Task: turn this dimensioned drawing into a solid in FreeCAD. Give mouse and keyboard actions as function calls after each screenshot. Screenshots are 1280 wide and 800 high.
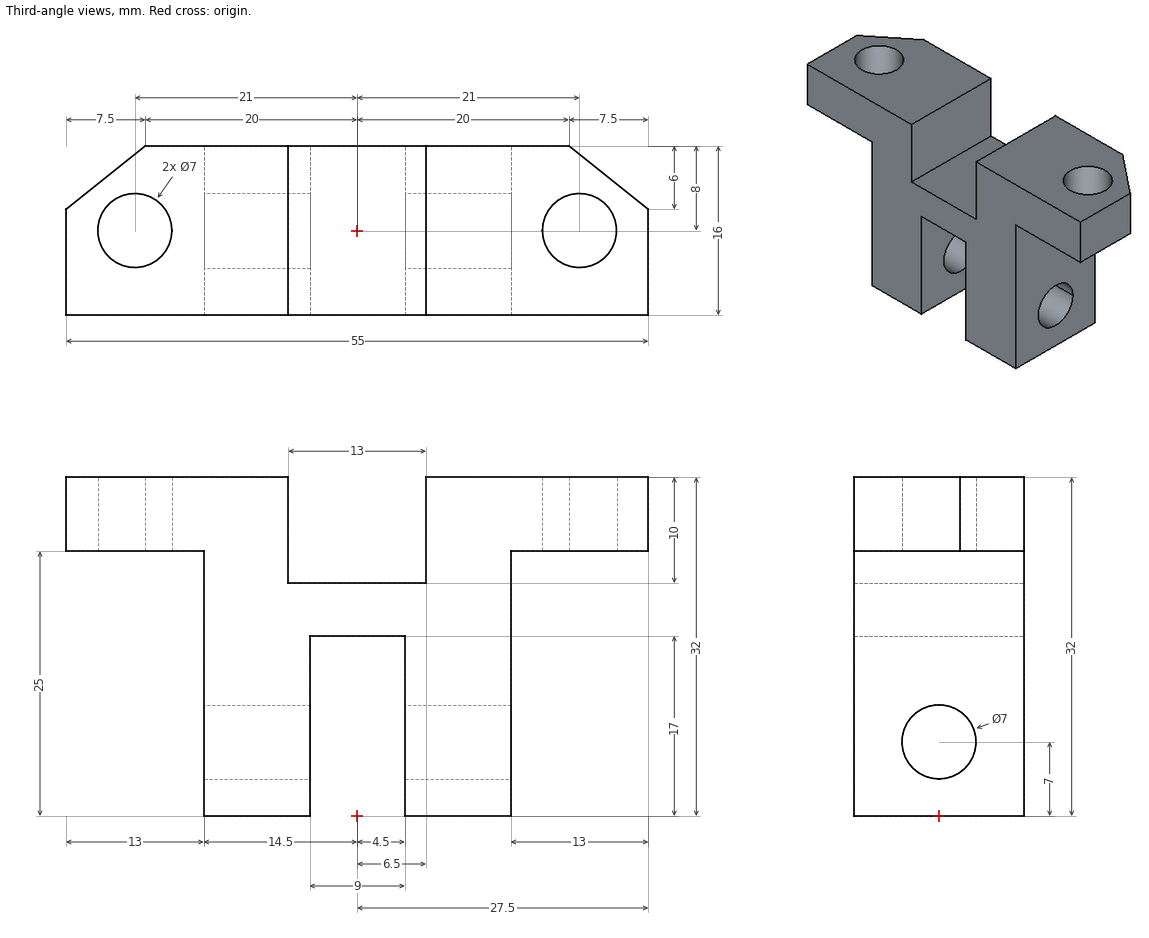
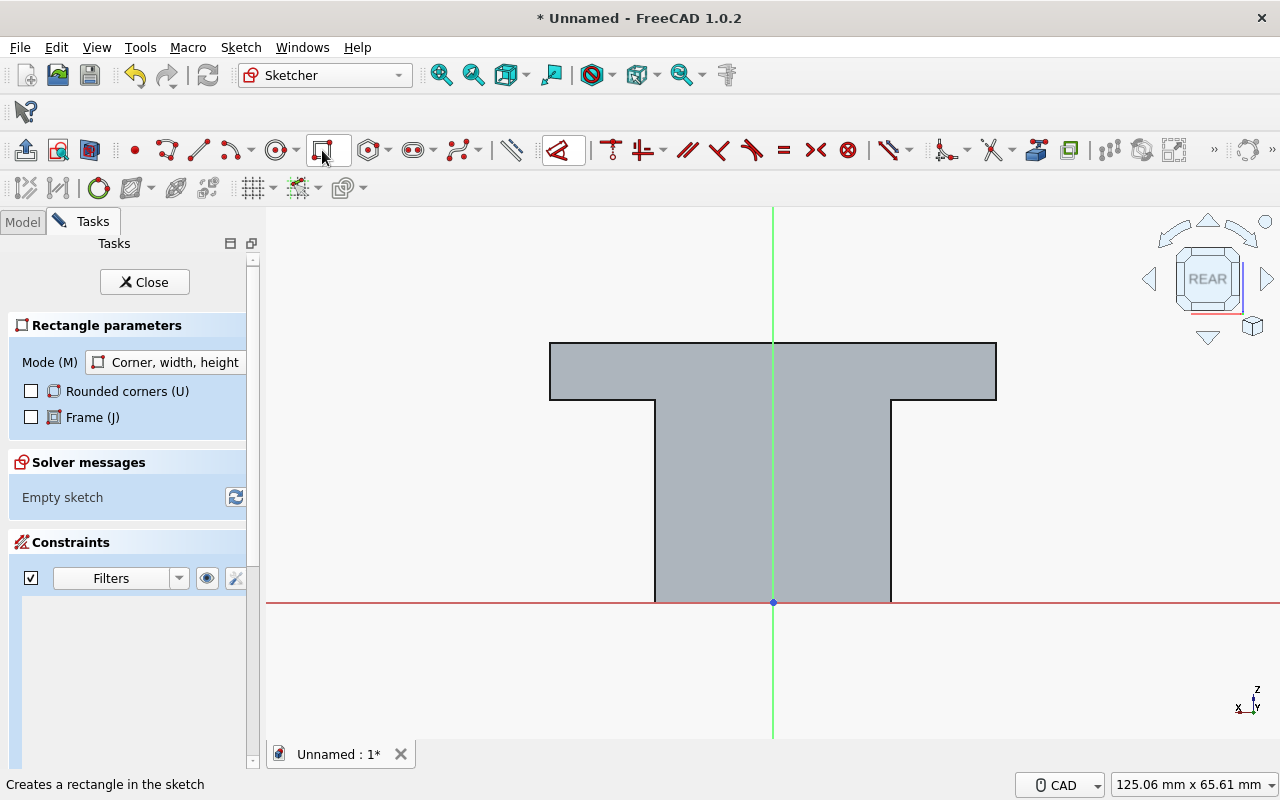
click(720, 343)
click(826, 424)
key(Escape)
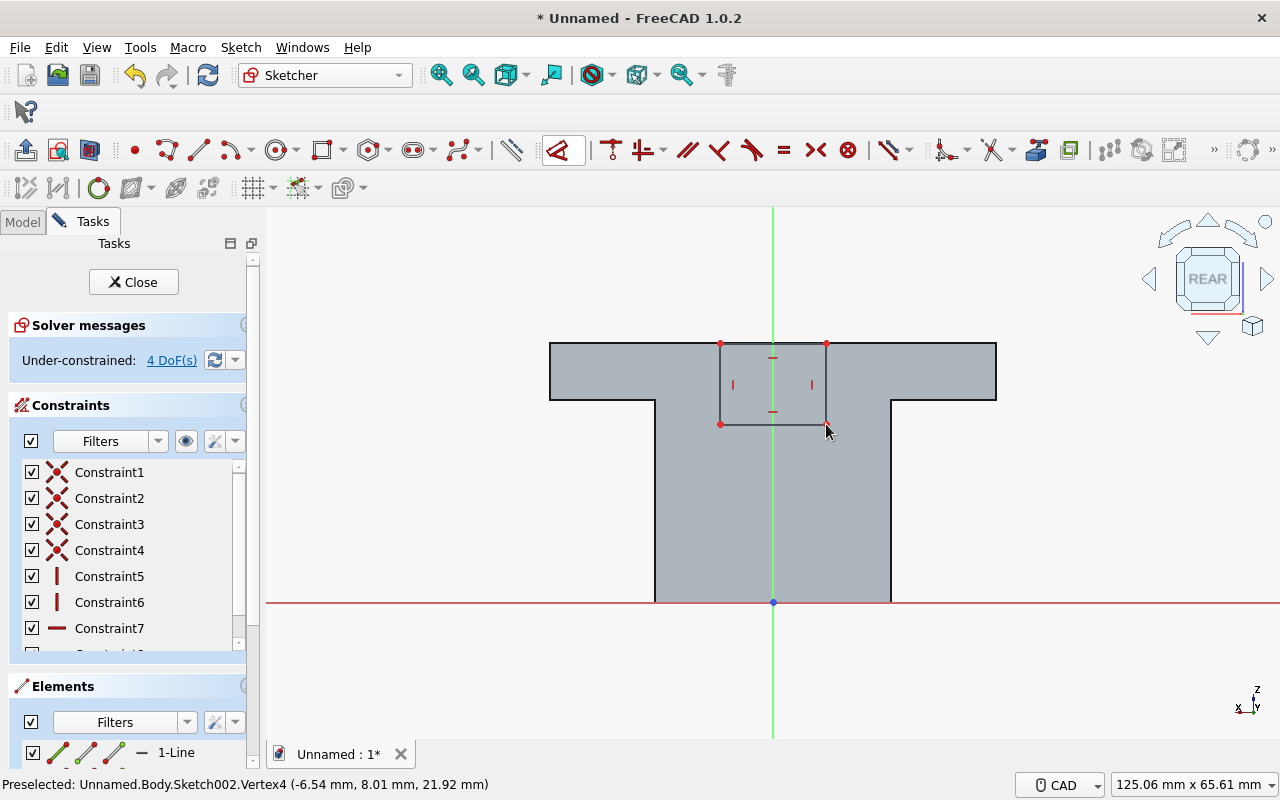
click(720, 368)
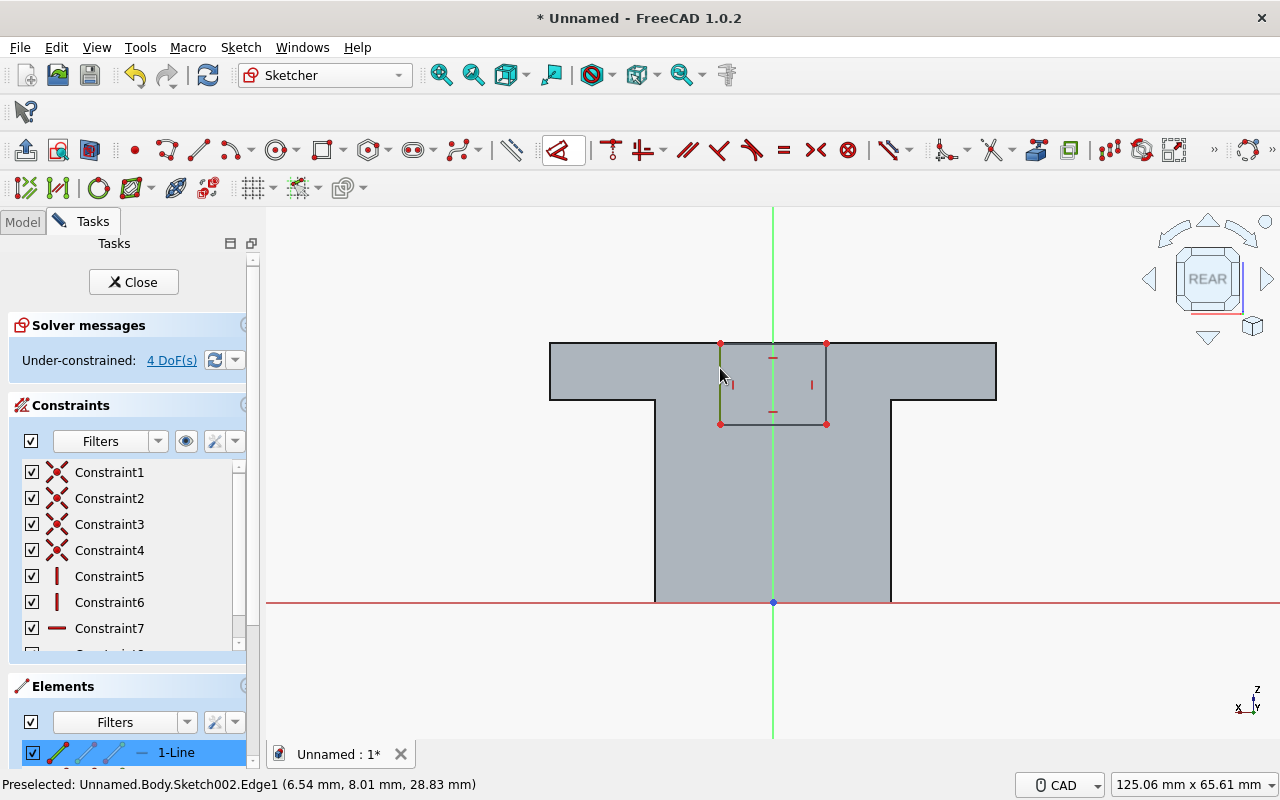
key(i)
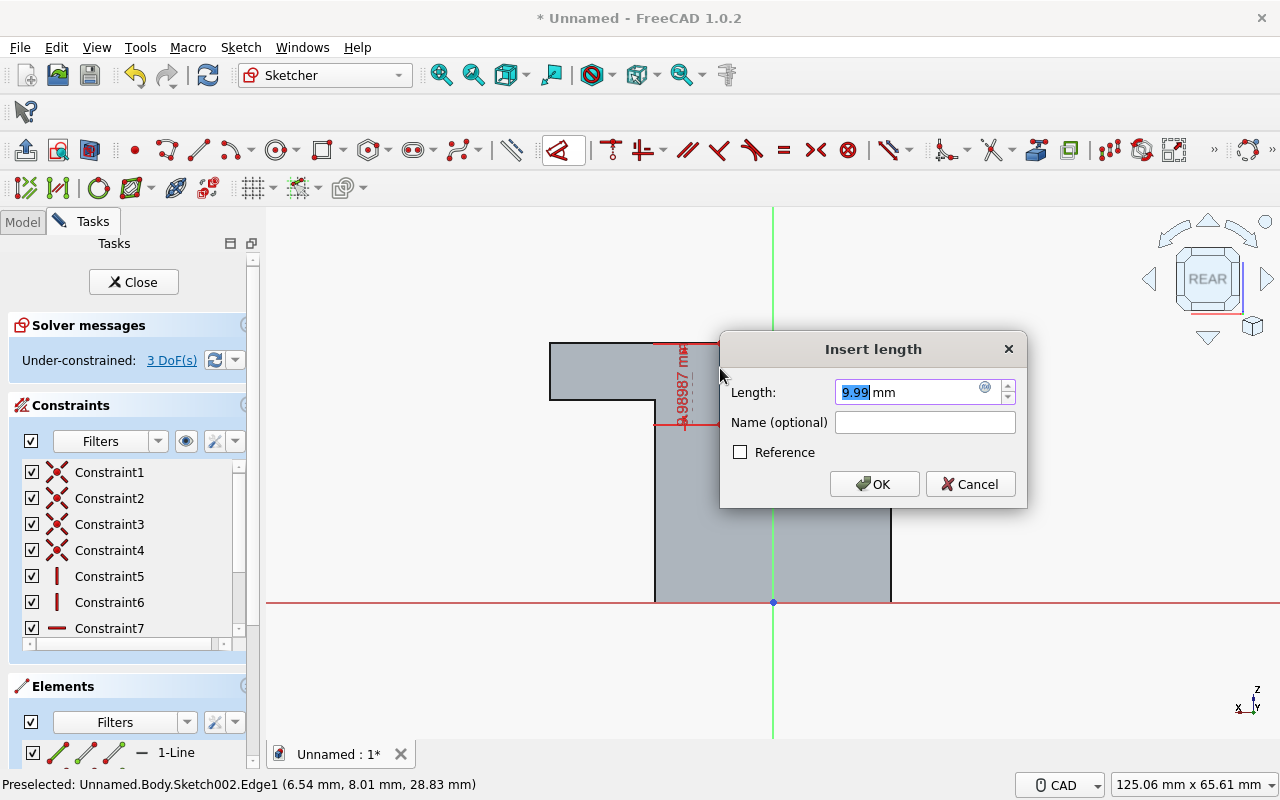
text(10)
key(Return)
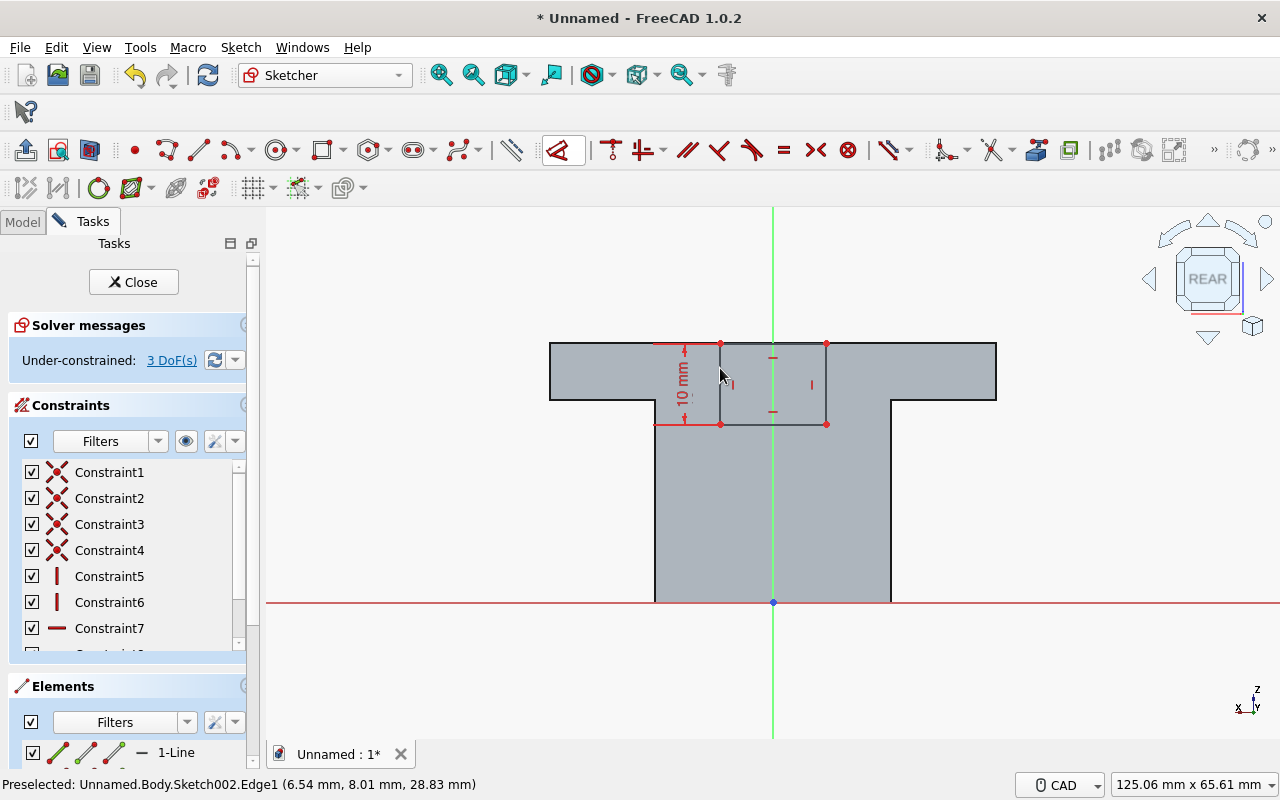
click(752, 425)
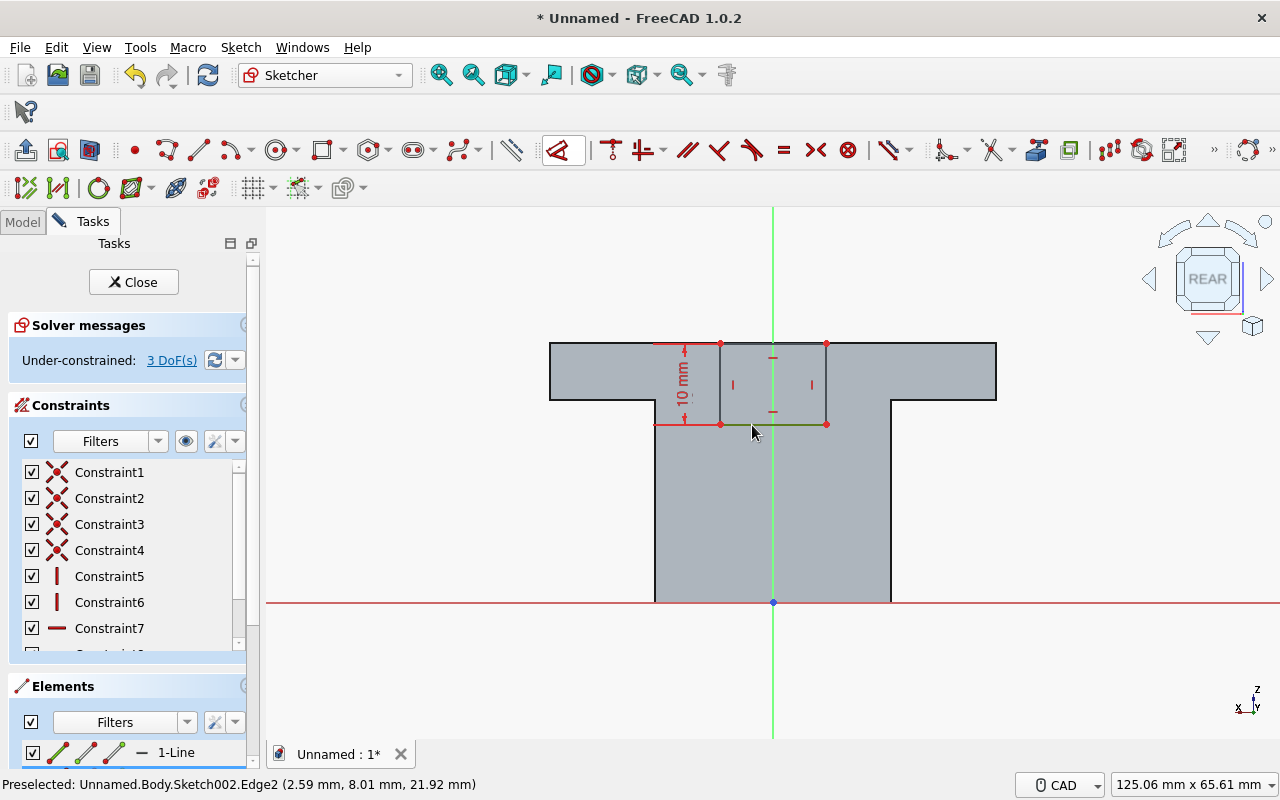
click(580, 150)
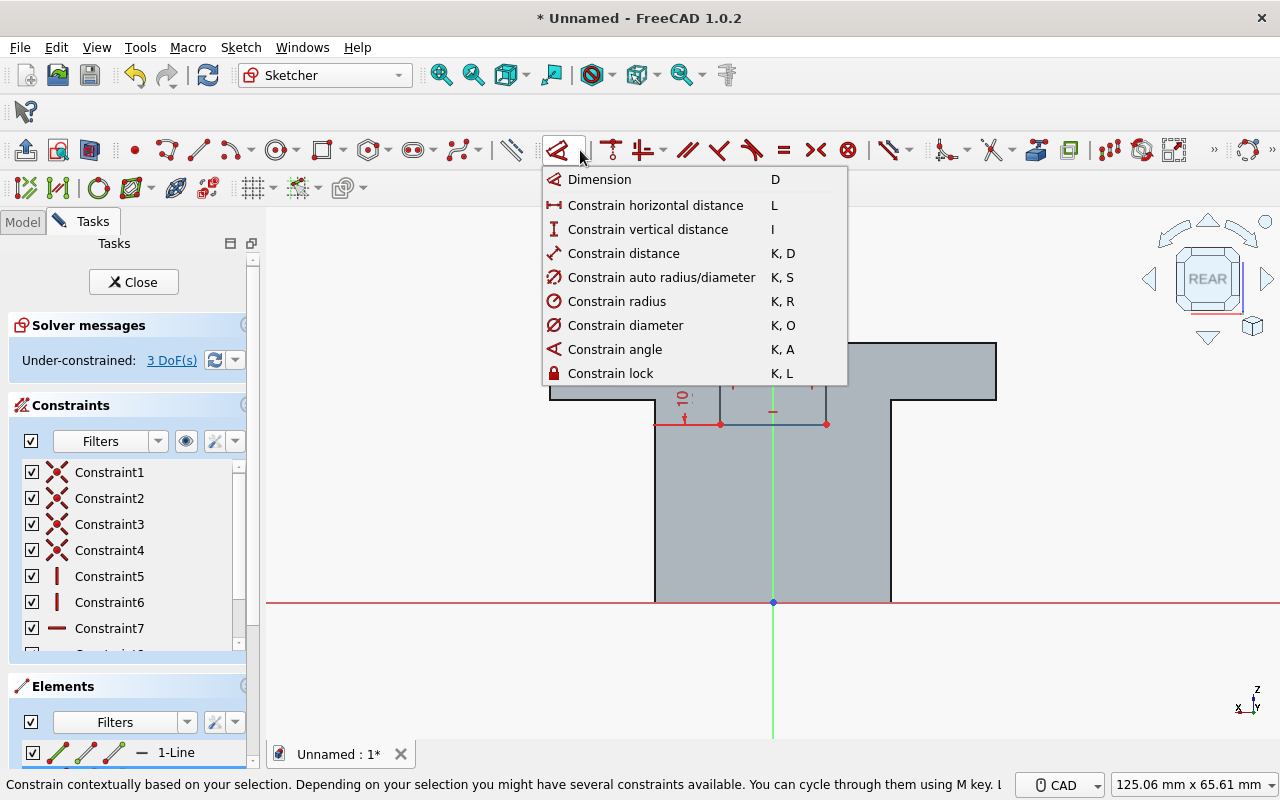
click(695, 205)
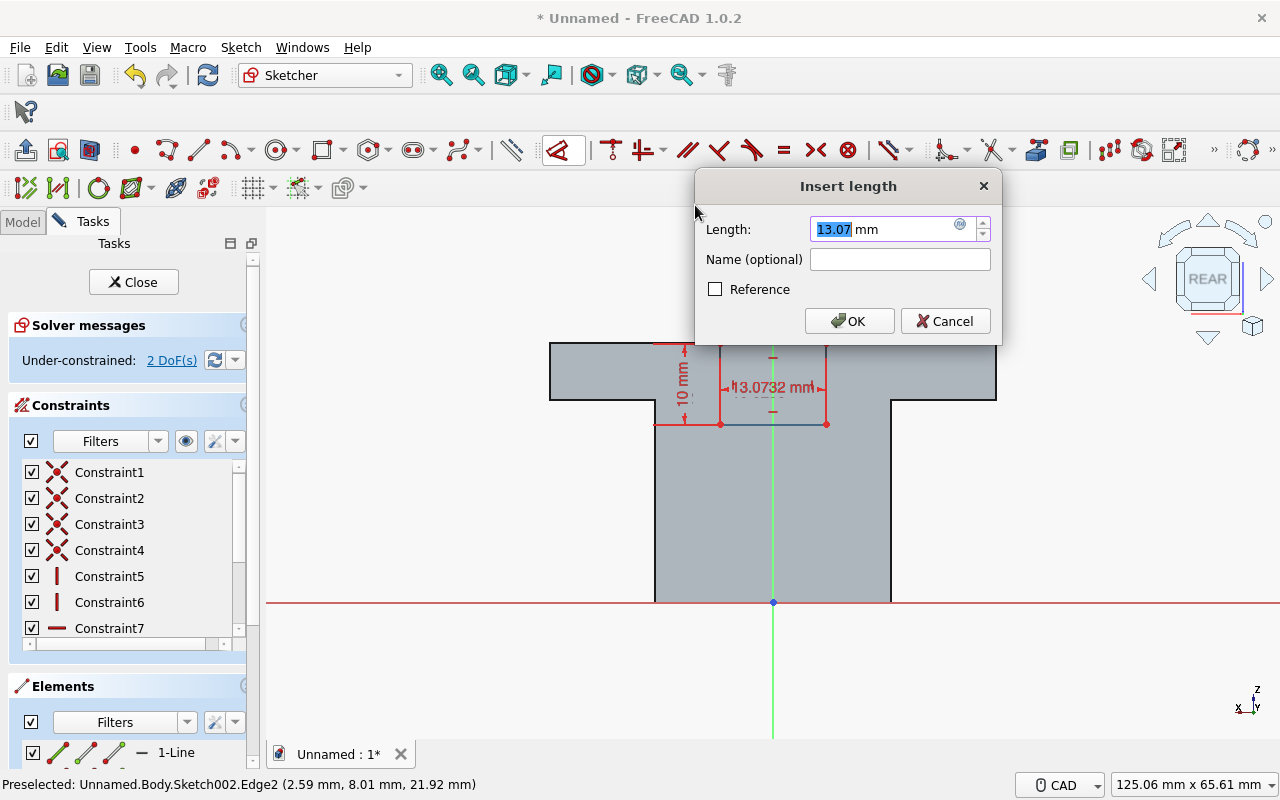
text(13)
key(Return)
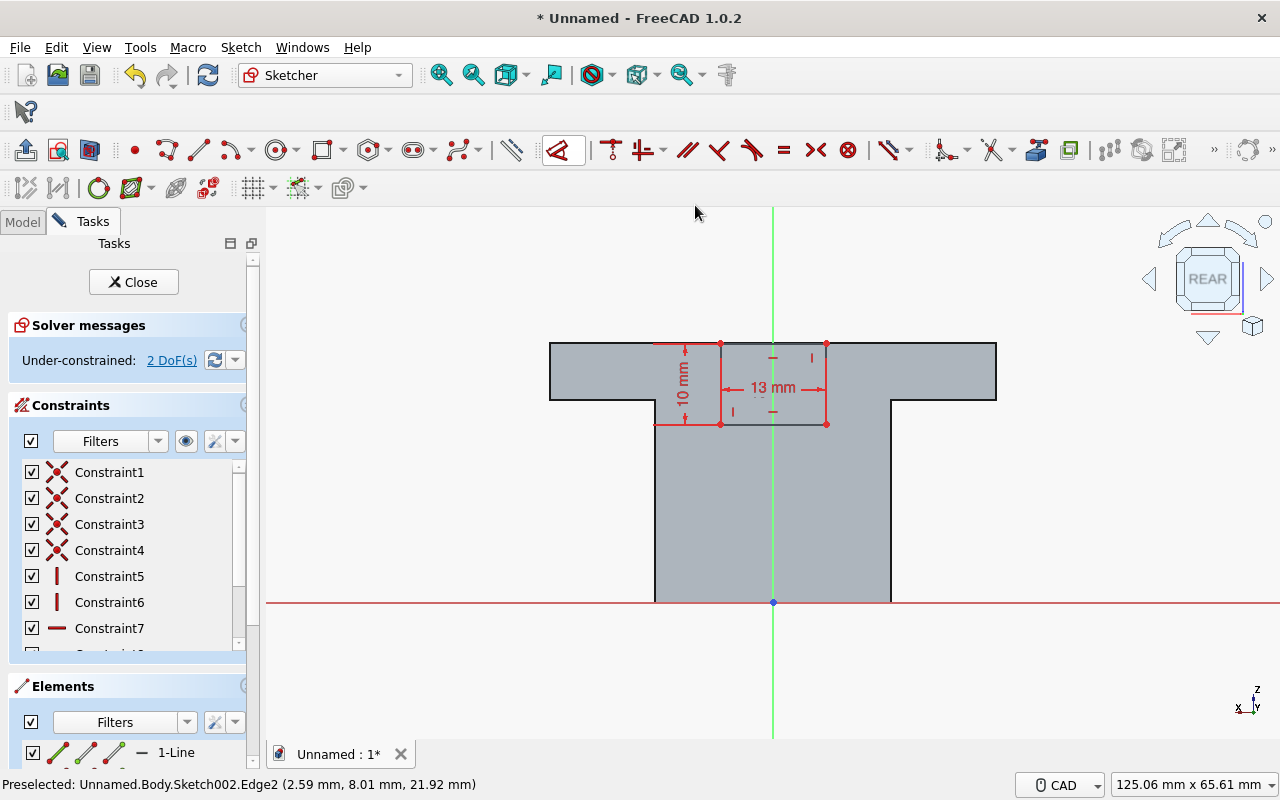
click(721, 344)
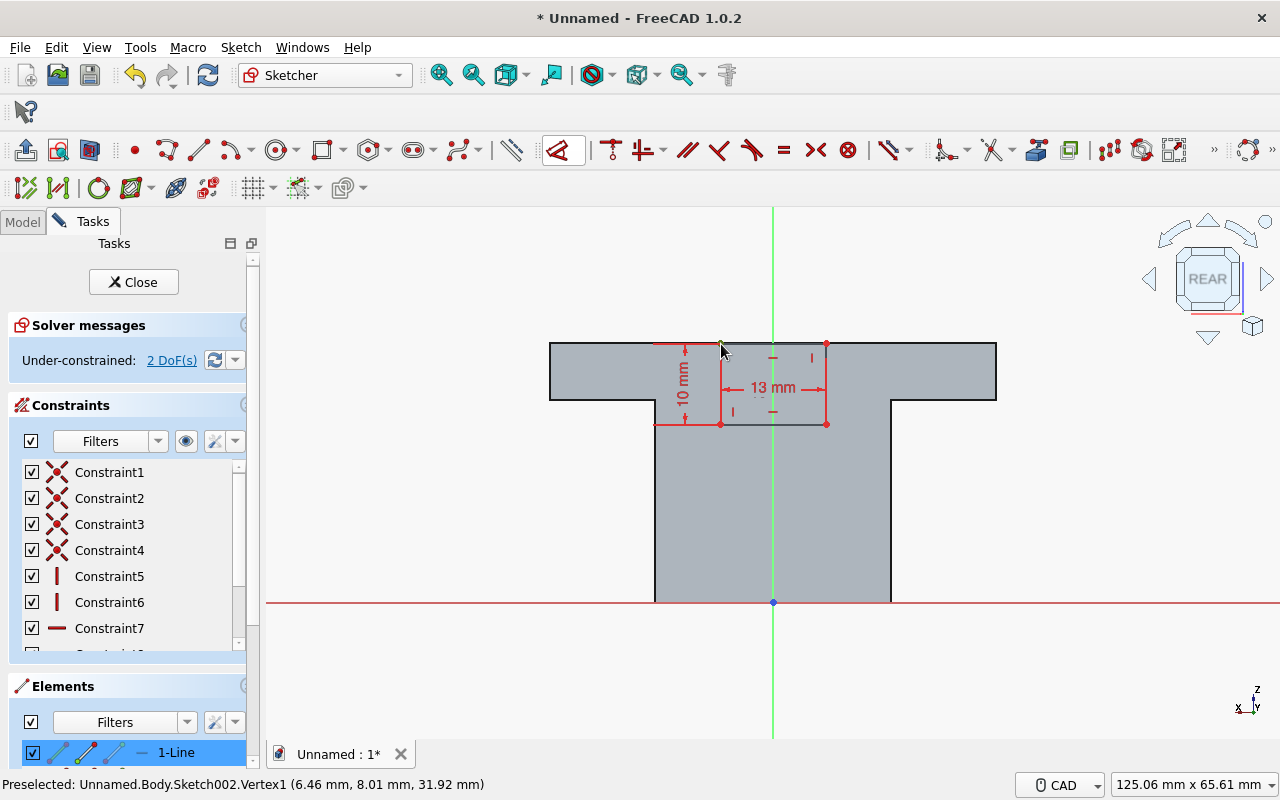
key(i)